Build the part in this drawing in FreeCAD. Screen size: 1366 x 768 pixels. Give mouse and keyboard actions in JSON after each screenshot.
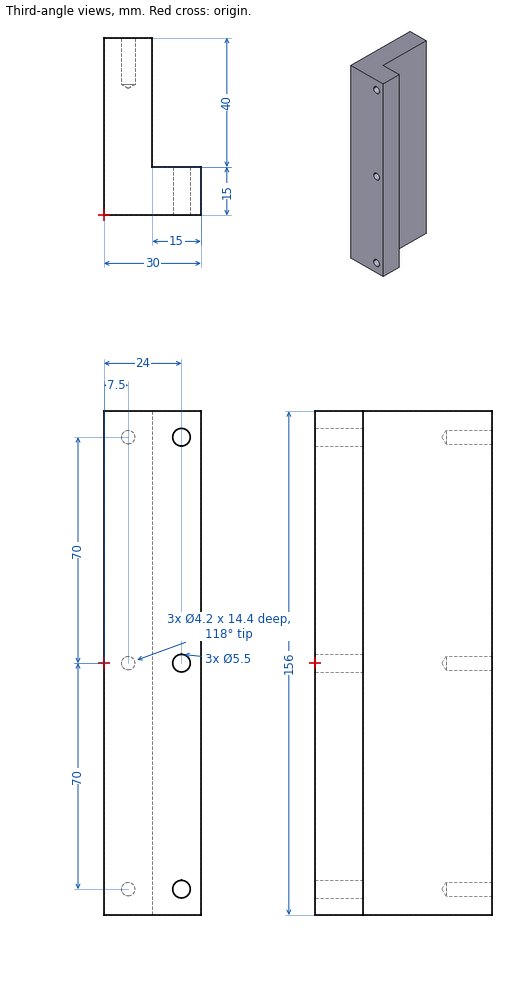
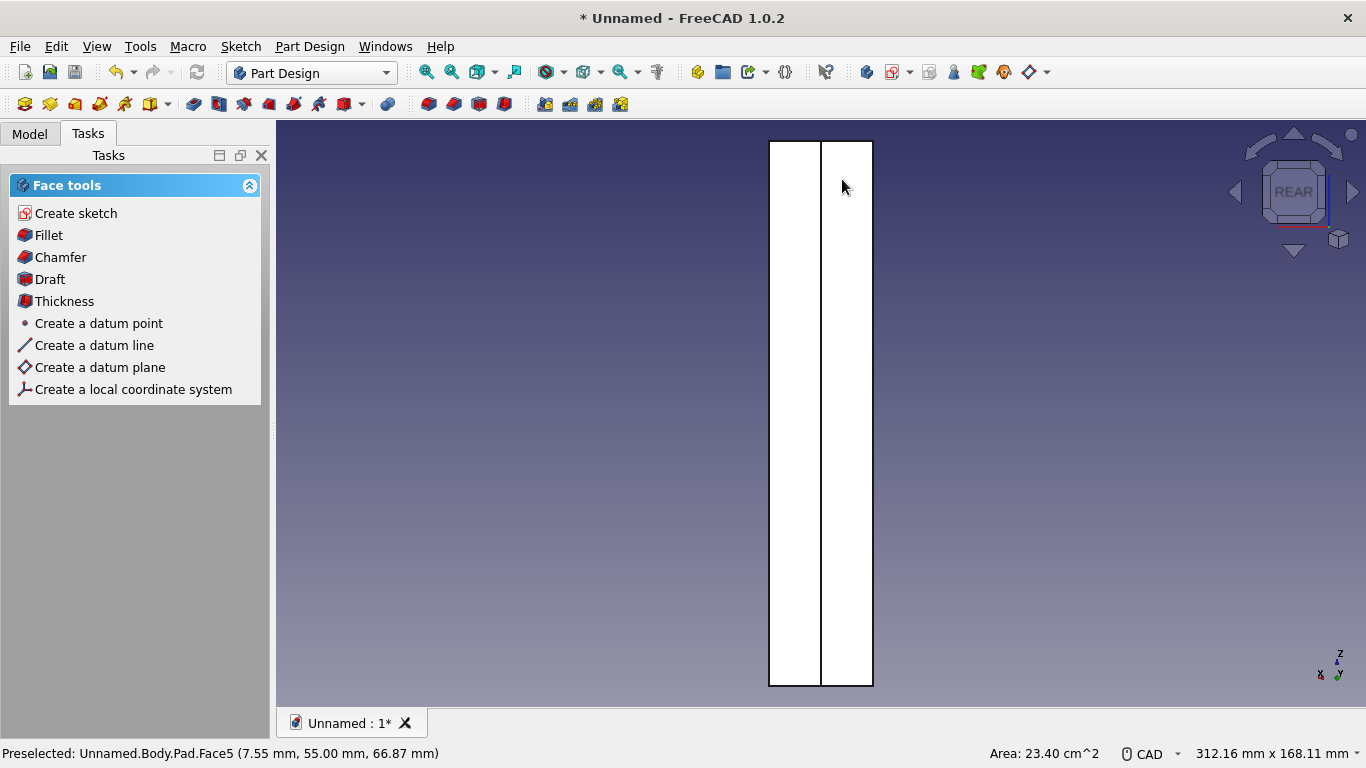
{"action": "left_click", "coordinate": [892, 72]}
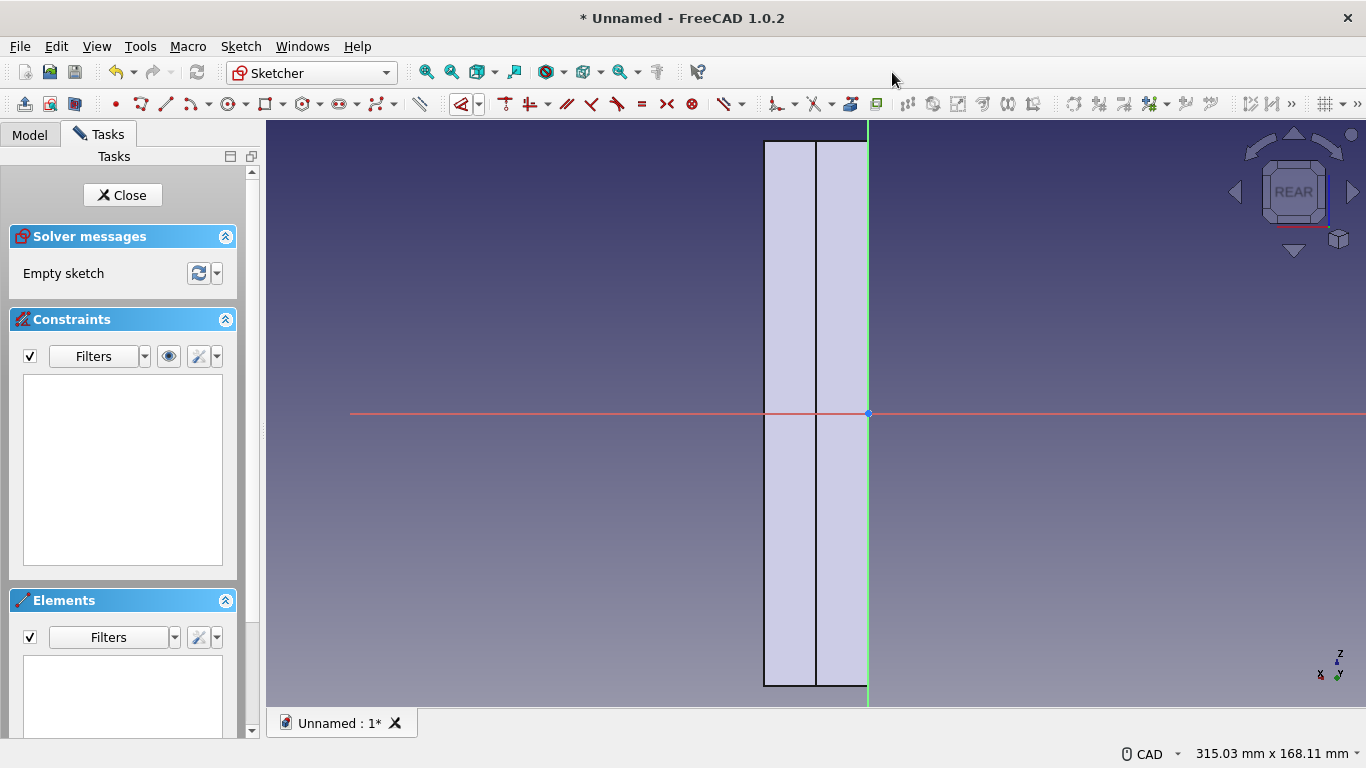
{"action": "scroll", "coordinate": [294, 414], "scroll_direction": "down", "scroll_amount": 1}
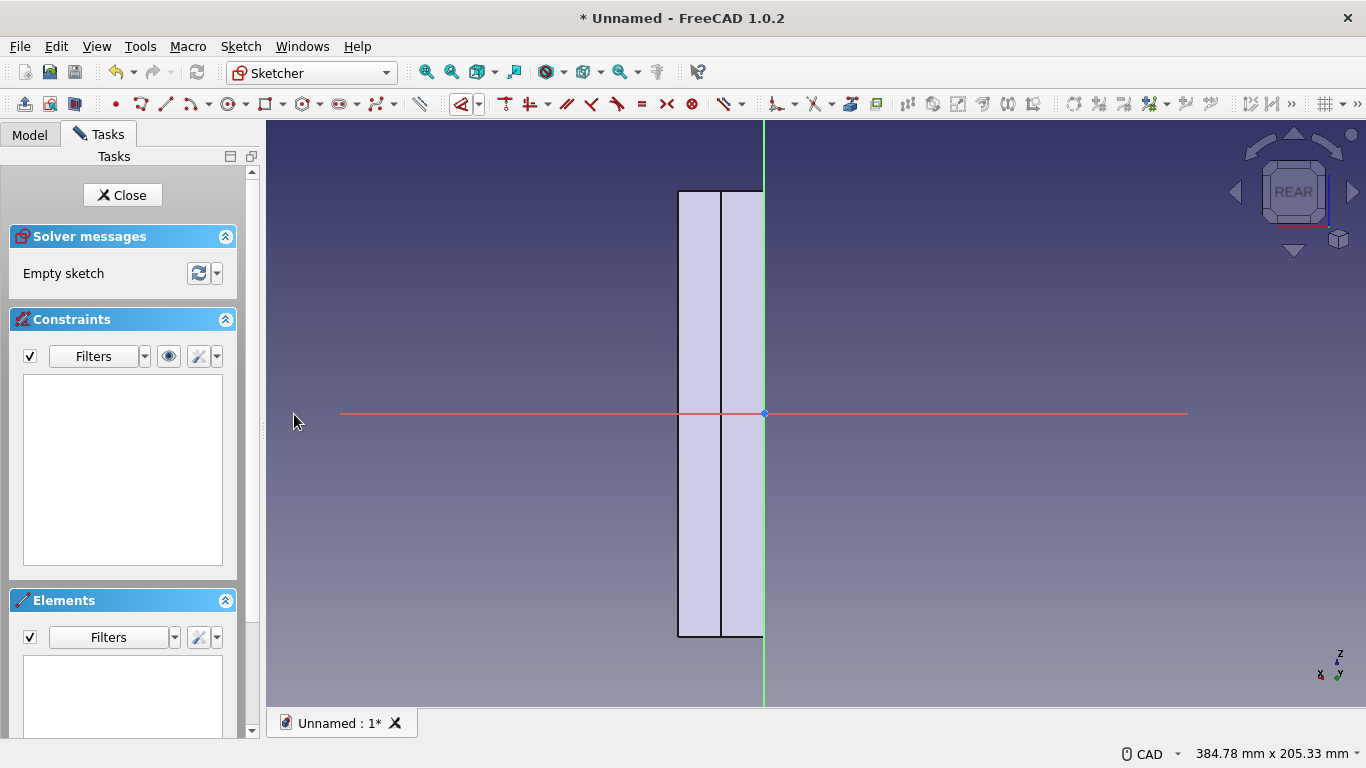
{"action": "key", "text": "g c"}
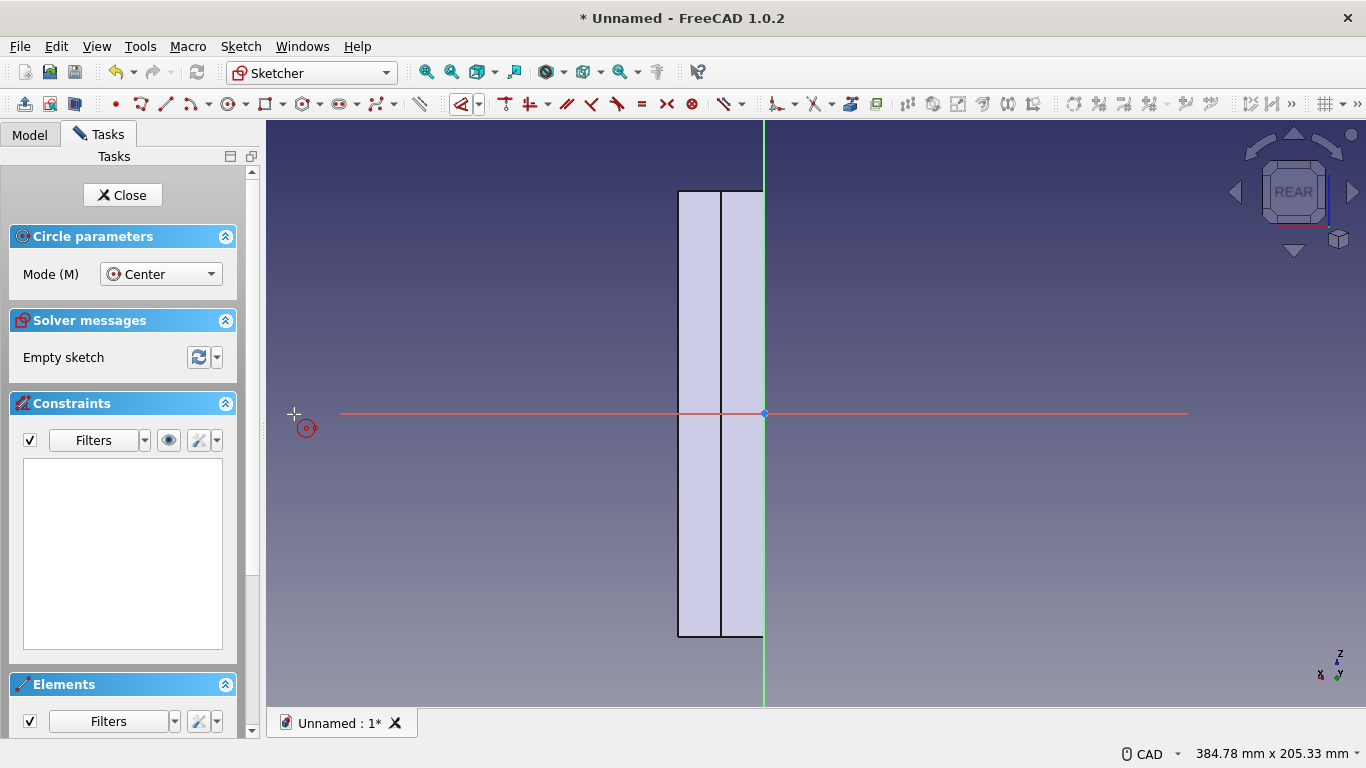
{"action": "scroll", "coordinate": [743, 414], "scroll_direction": "up", "scroll_amount": 7}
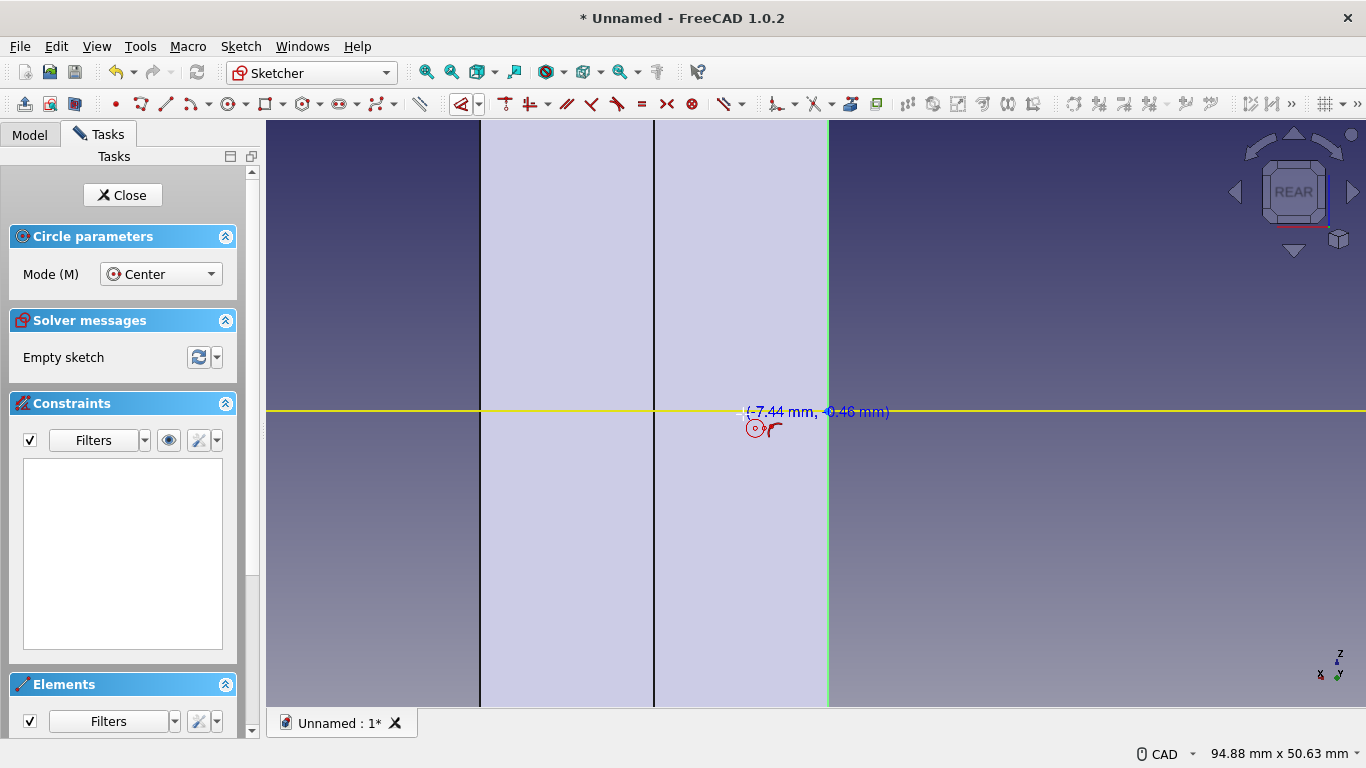
{"action": "scroll", "coordinate": [739, 414], "scroll_direction": "down", "scroll_amount": 7}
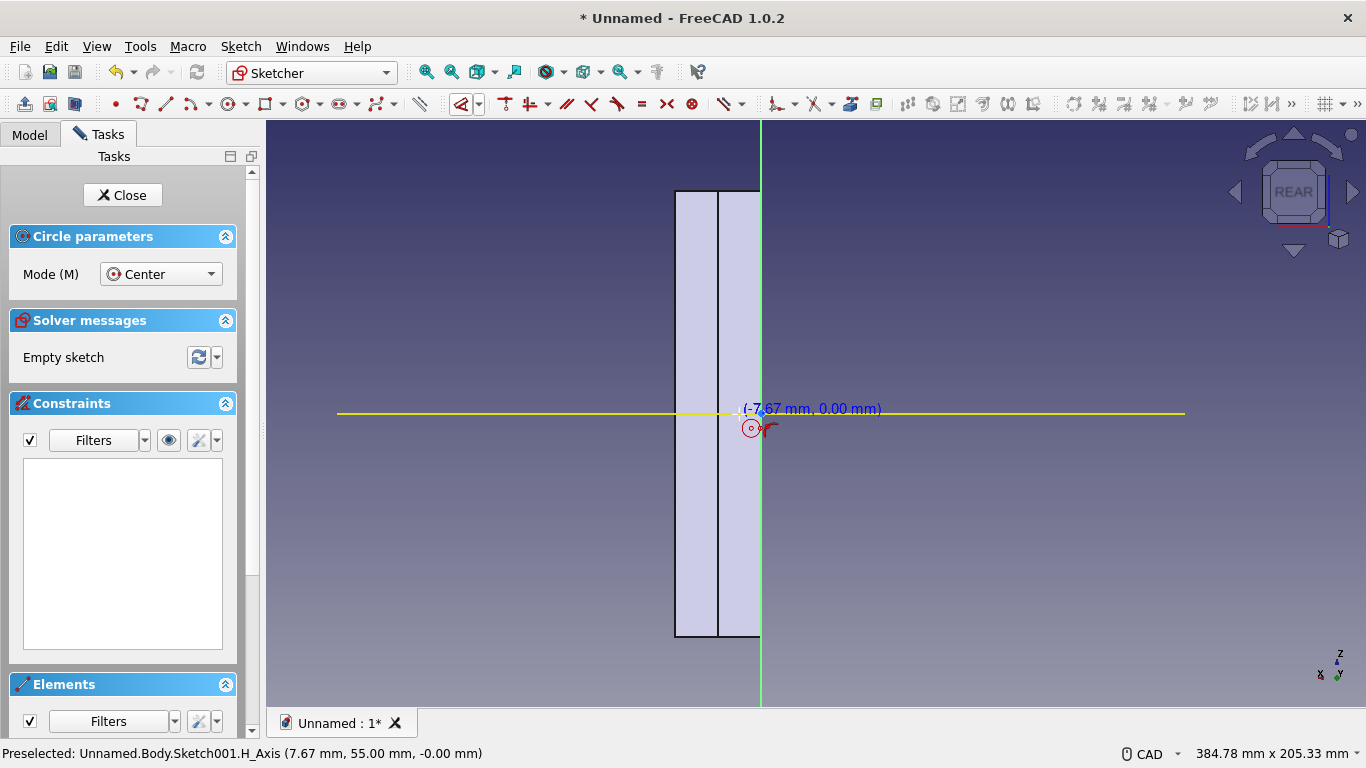
{"action": "left_click", "coordinate": [740, 414]}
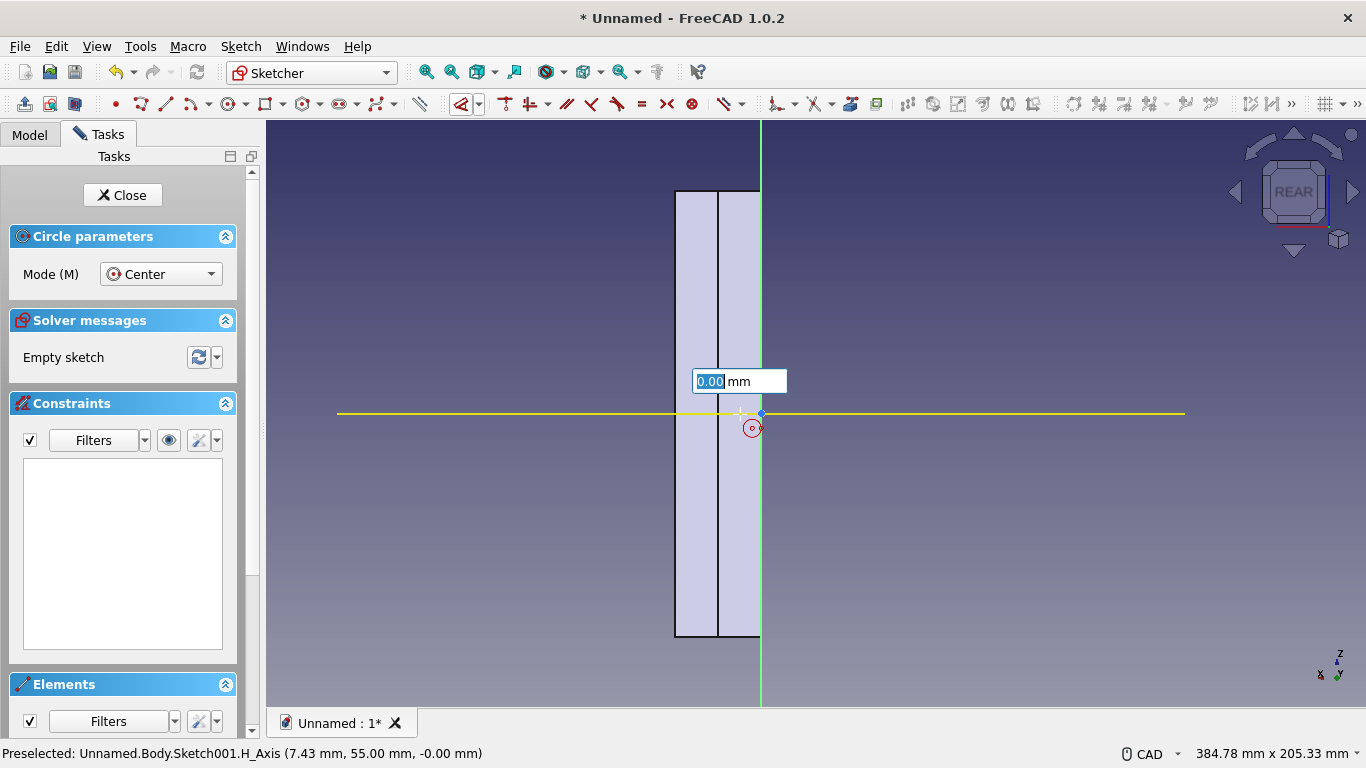
{"action": "scroll", "coordinate": [742, 408], "scroll_direction": "up", "scroll_amount": 6}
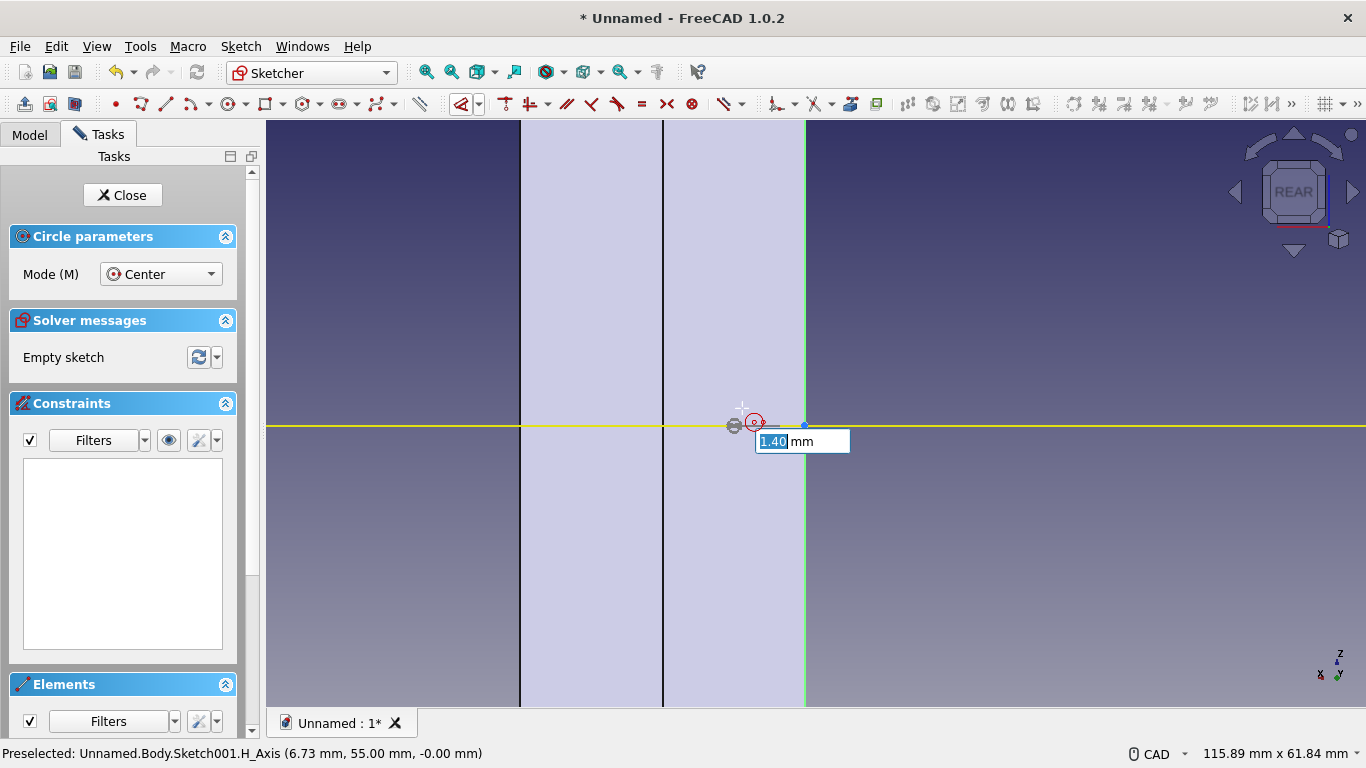
{"action": "left_click", "coordinate": [741, 407]}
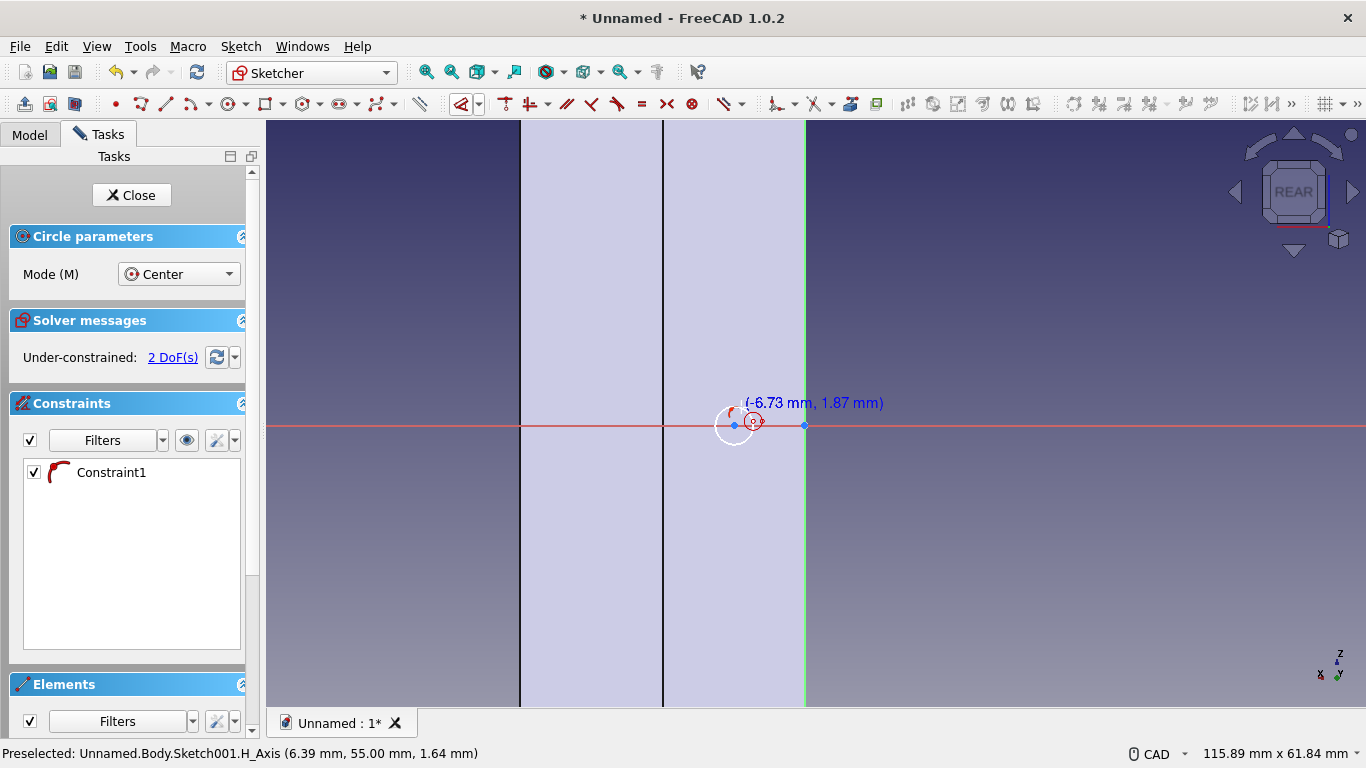
{"action": "scroll", "coordinate": [742, 408], "scroll_direction": "down", "scroll_amount": 6}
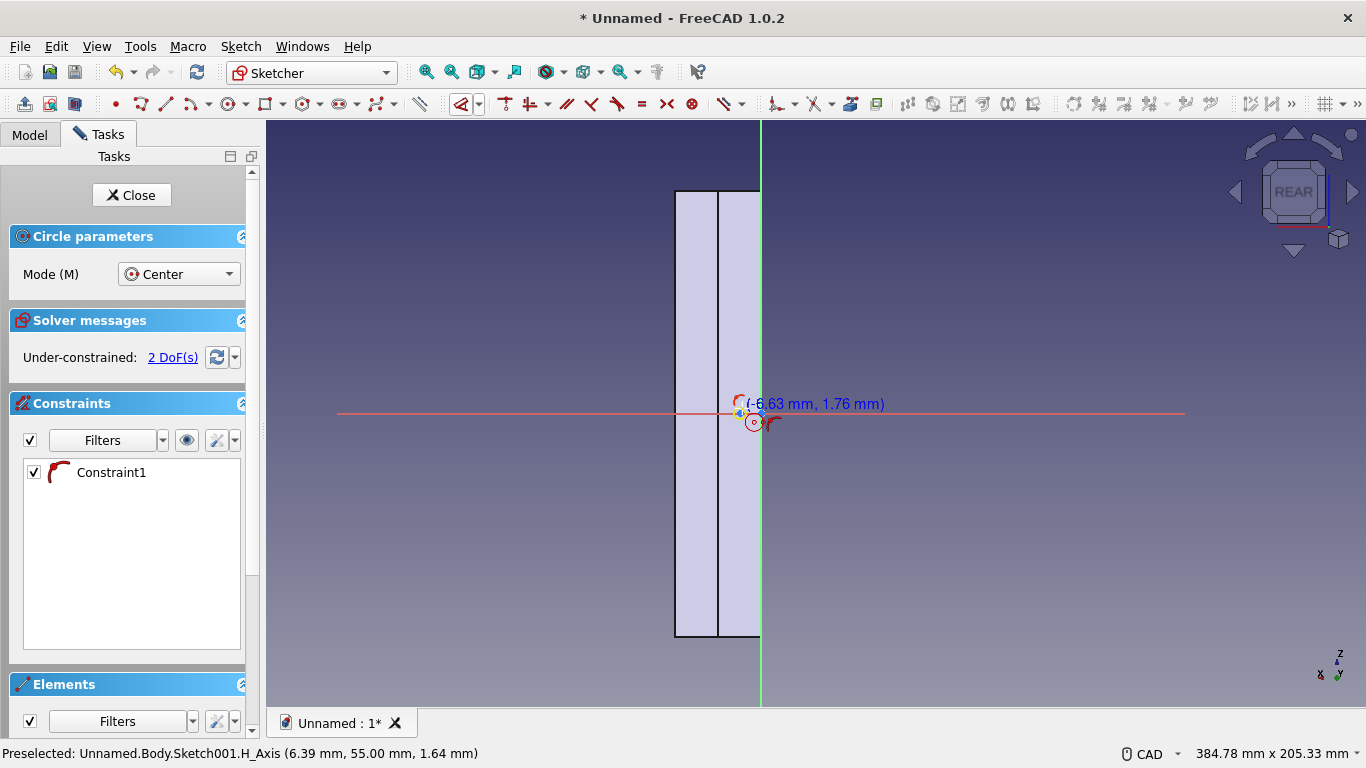
{"action": "scroll", "coordinate": [740, 614], "scroll_direction": "up", "scroll_amount": 7}